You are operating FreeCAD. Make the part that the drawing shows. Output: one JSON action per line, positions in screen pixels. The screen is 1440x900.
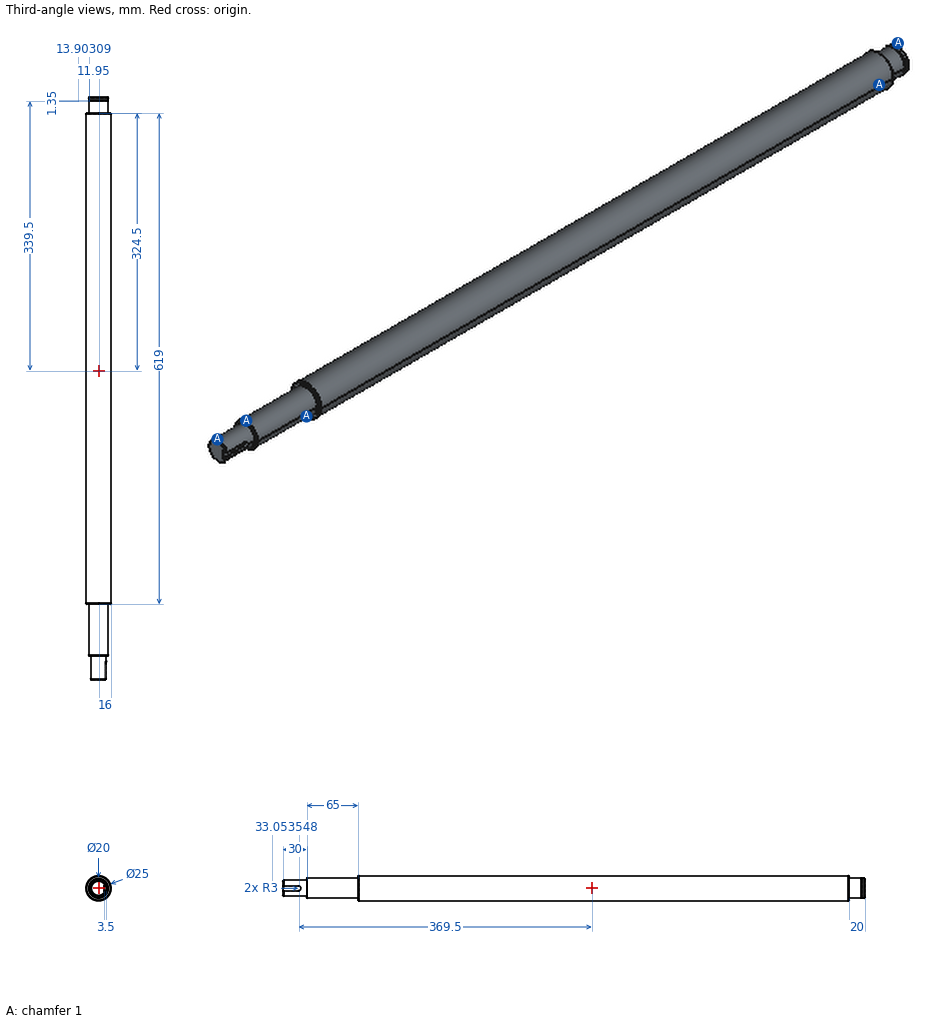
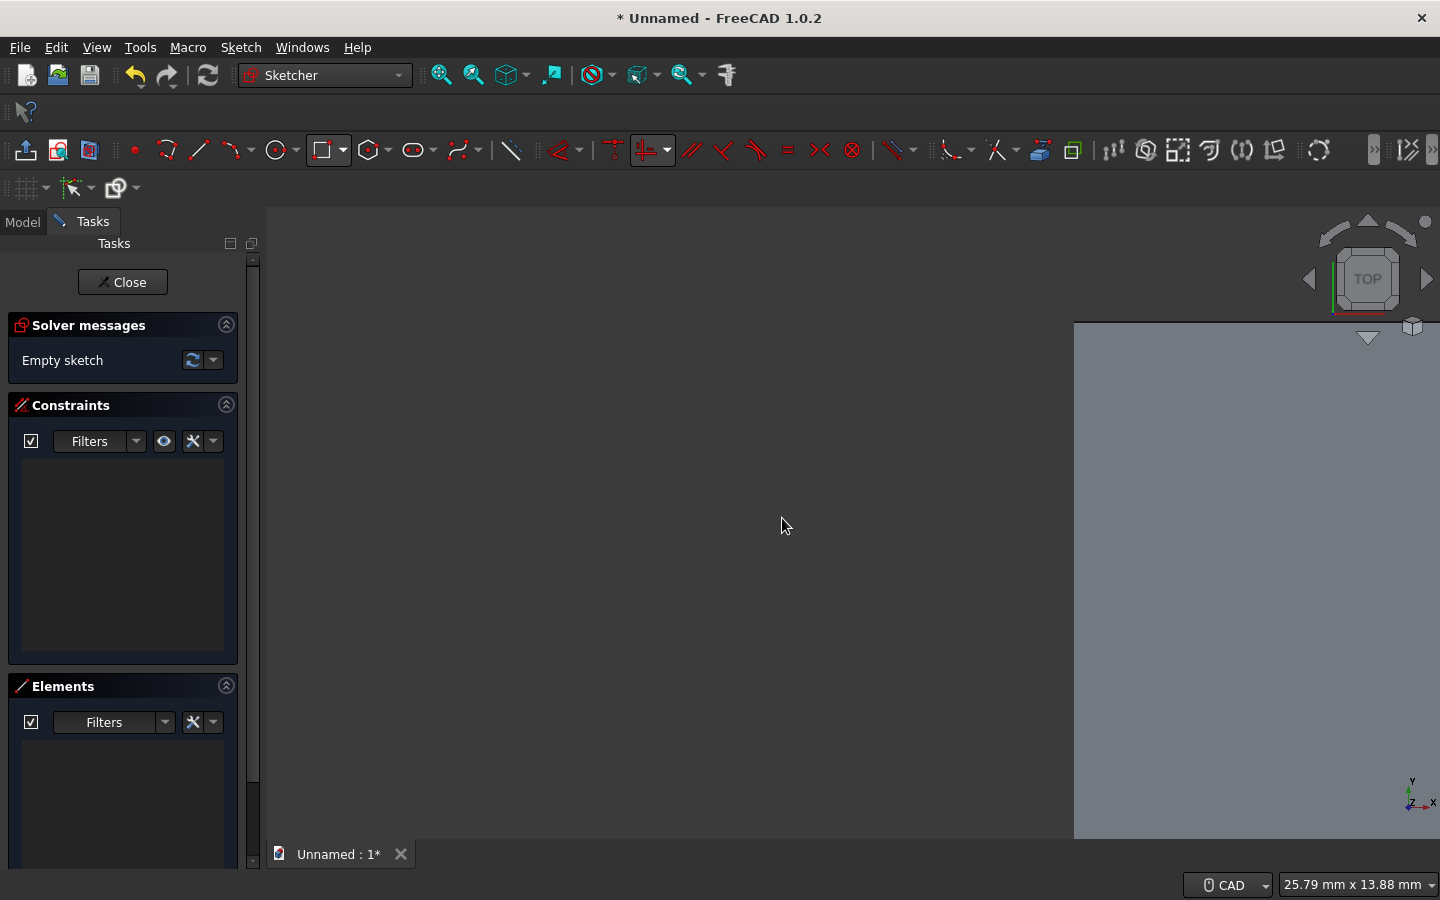
{"action": "left_click", "coordinate": [322, 150]}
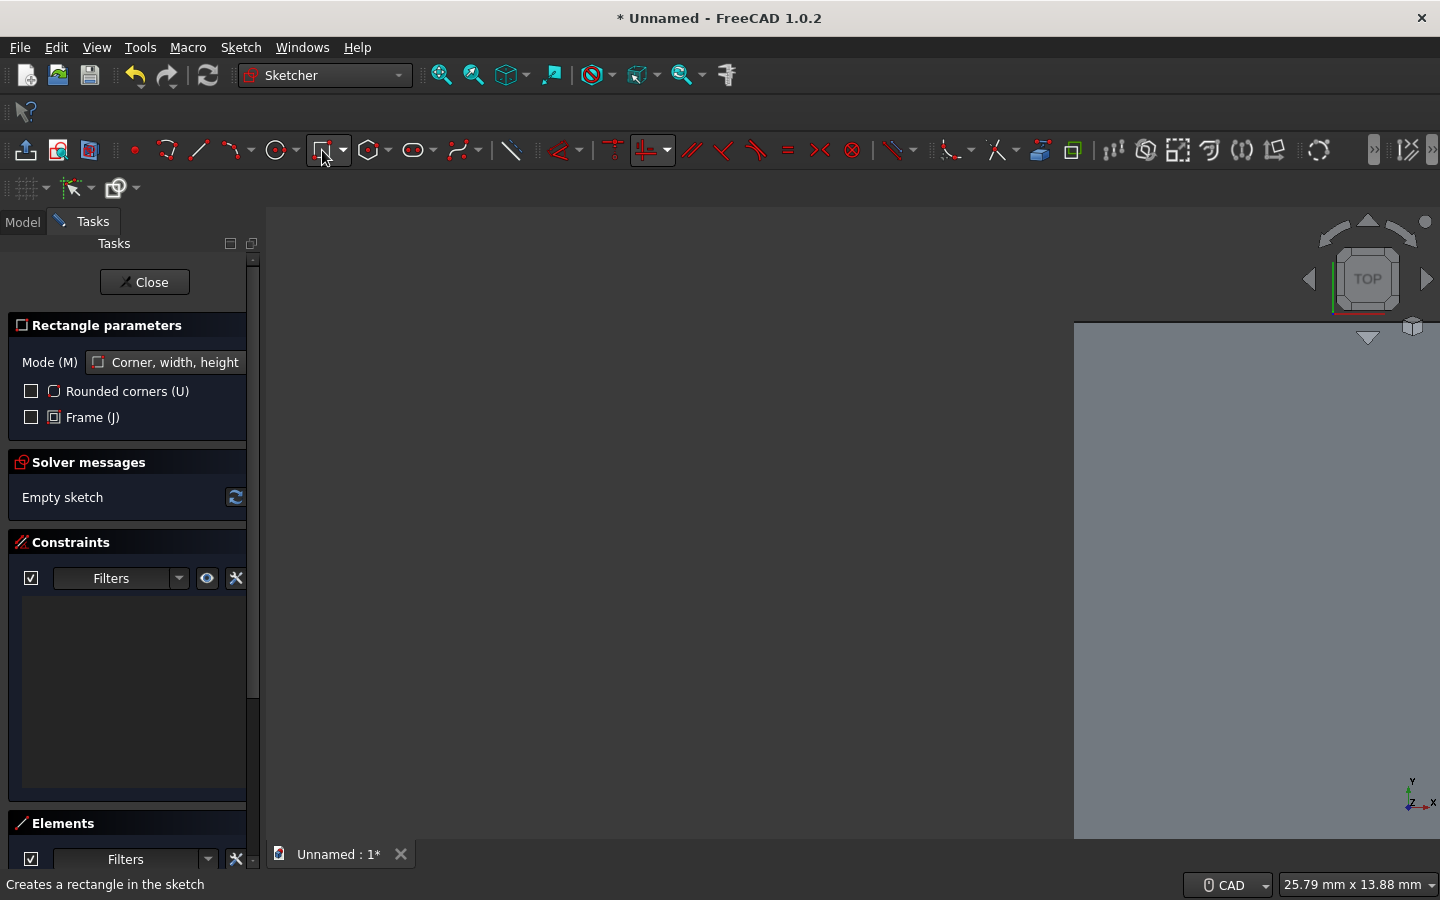
{"action": "left_click", "coordinate": [466, 488]}
{"action": "mouse_move", "coordinate": [1099, 549]}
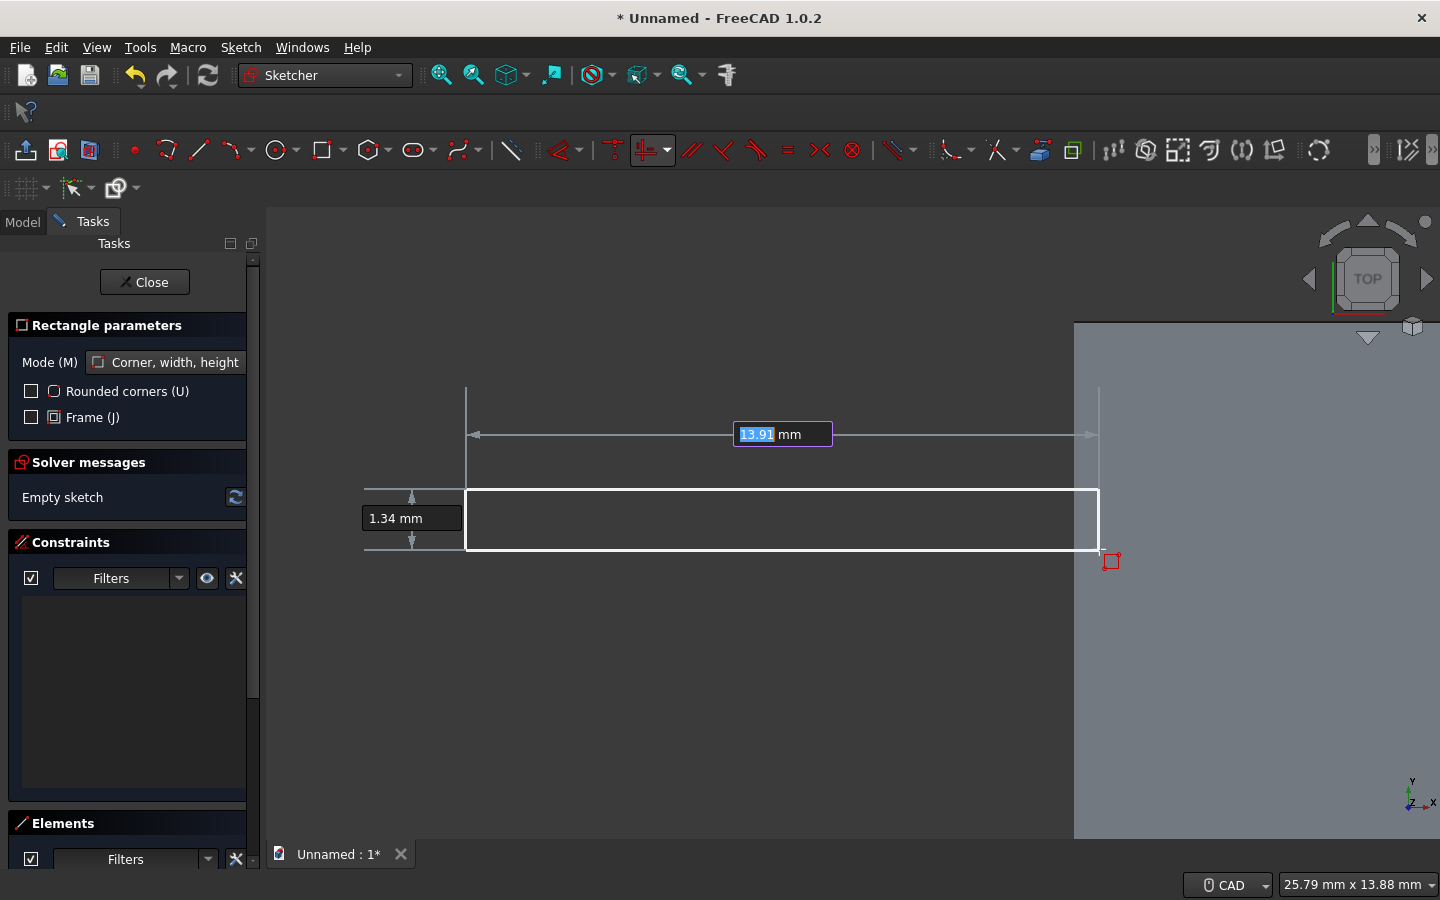
{"action": "type", "text": "13.90309"}
{"action": "key", "text": "Tab"}
{"action": "type", "text": "1.35"}
{"action": "key", "text": "Return"}
{"action": "key", "text": "Escape"}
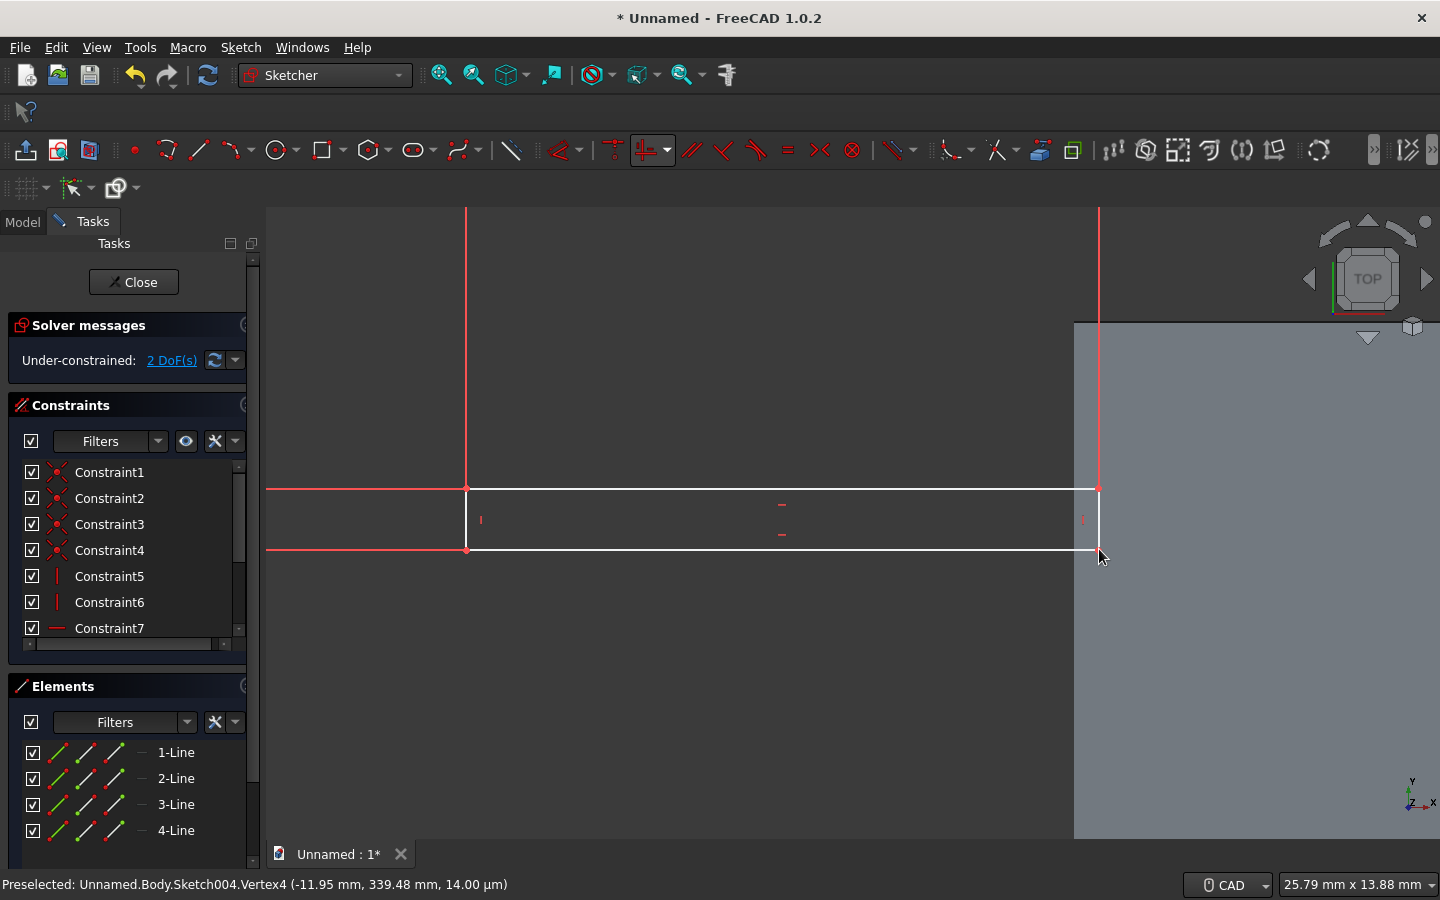
{"action": "left_click", "coordinate": [558, 150]}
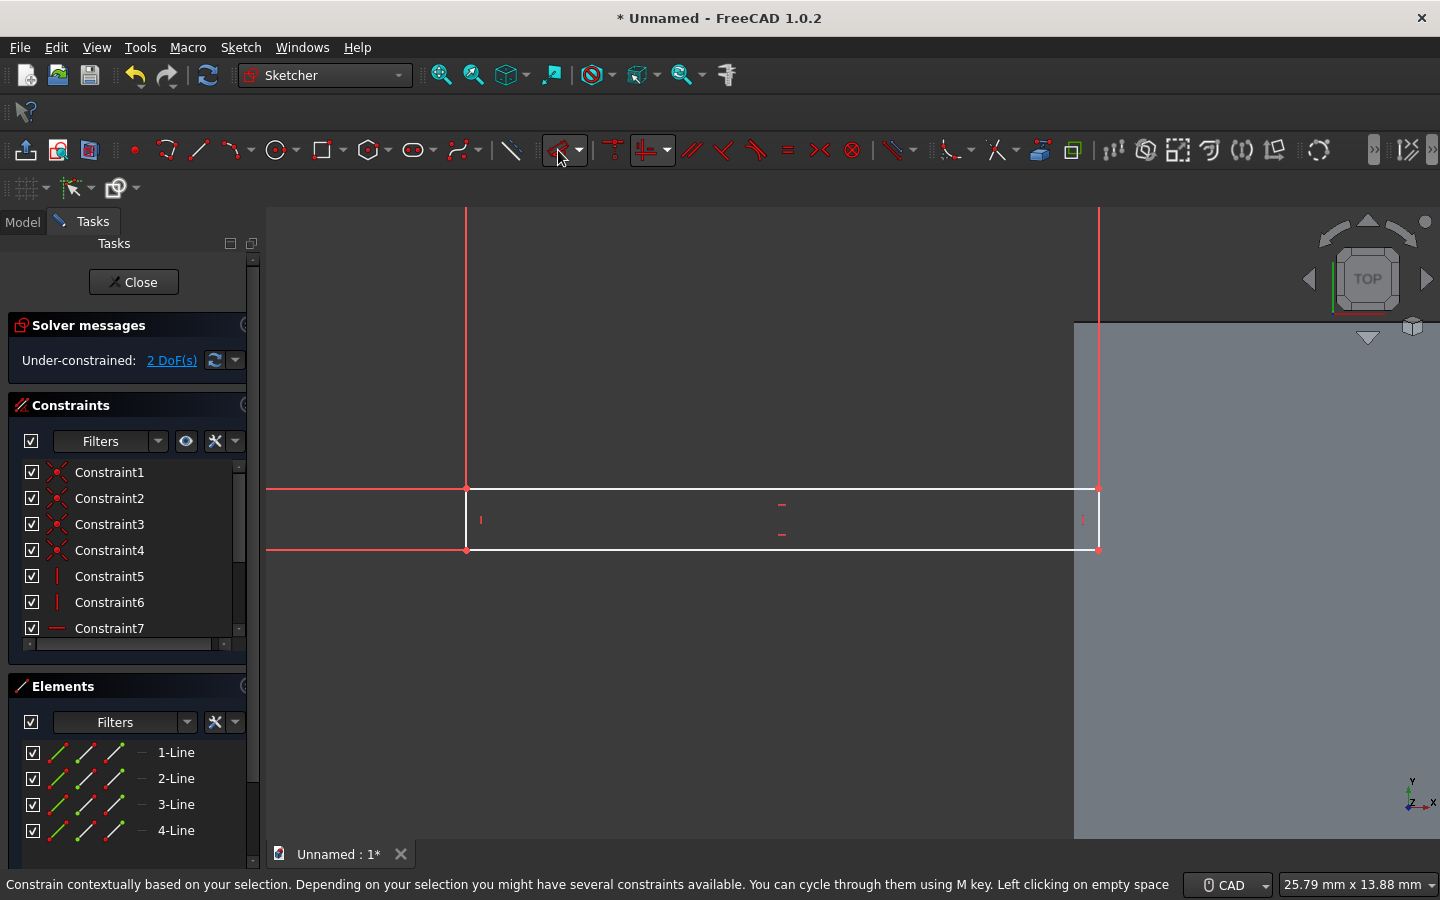
{"action": "left_click", "coordinate": [466, 550]}
{"action": "left_click", "coordinate": [432, 681]}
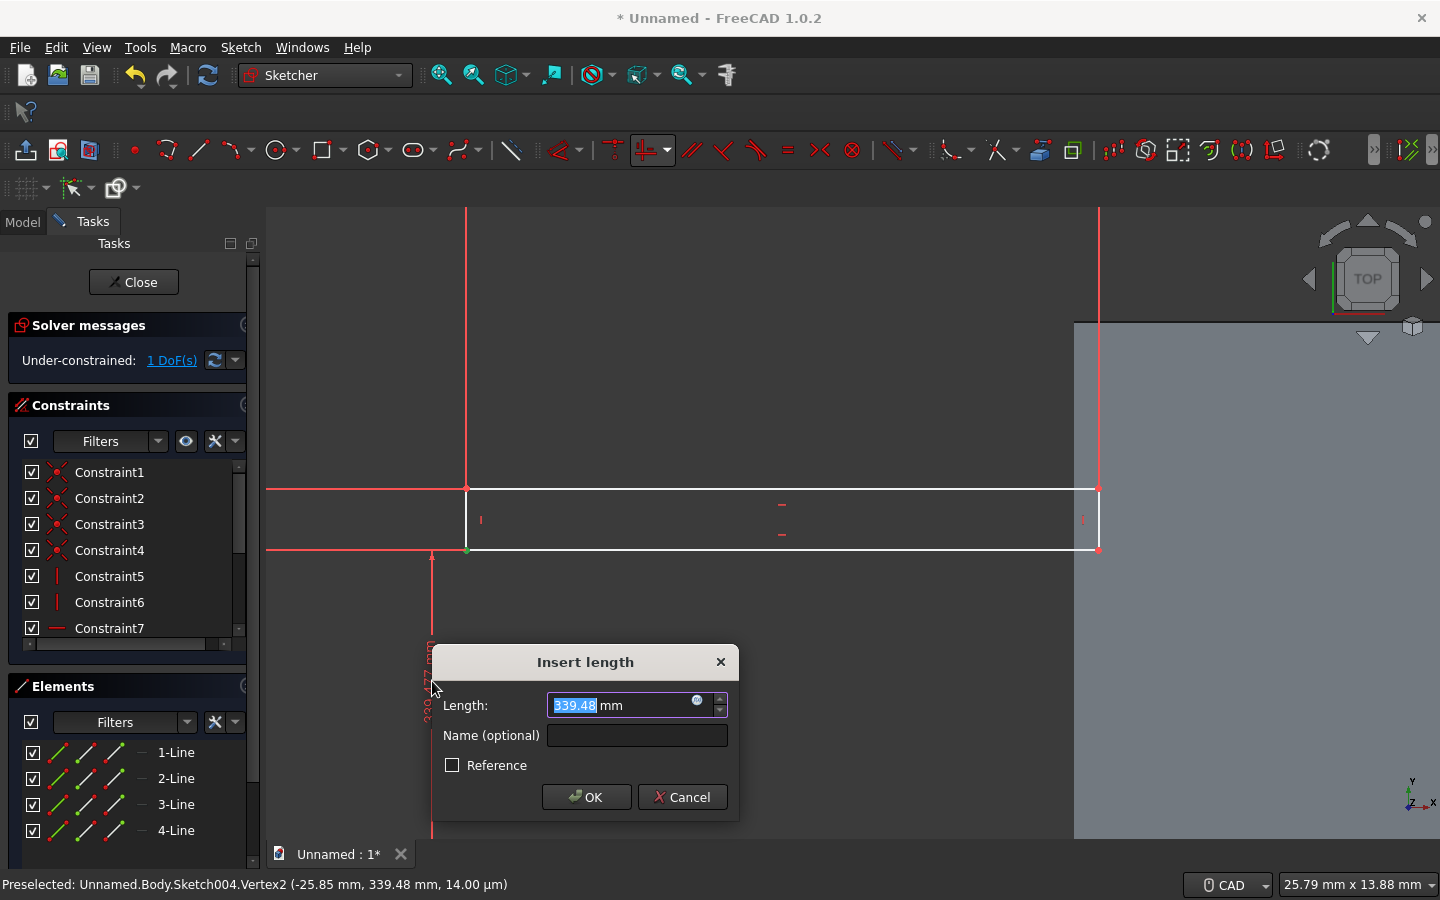
{"action": "type", "text": "339.5"}
{"action": "key", "text": "Return"}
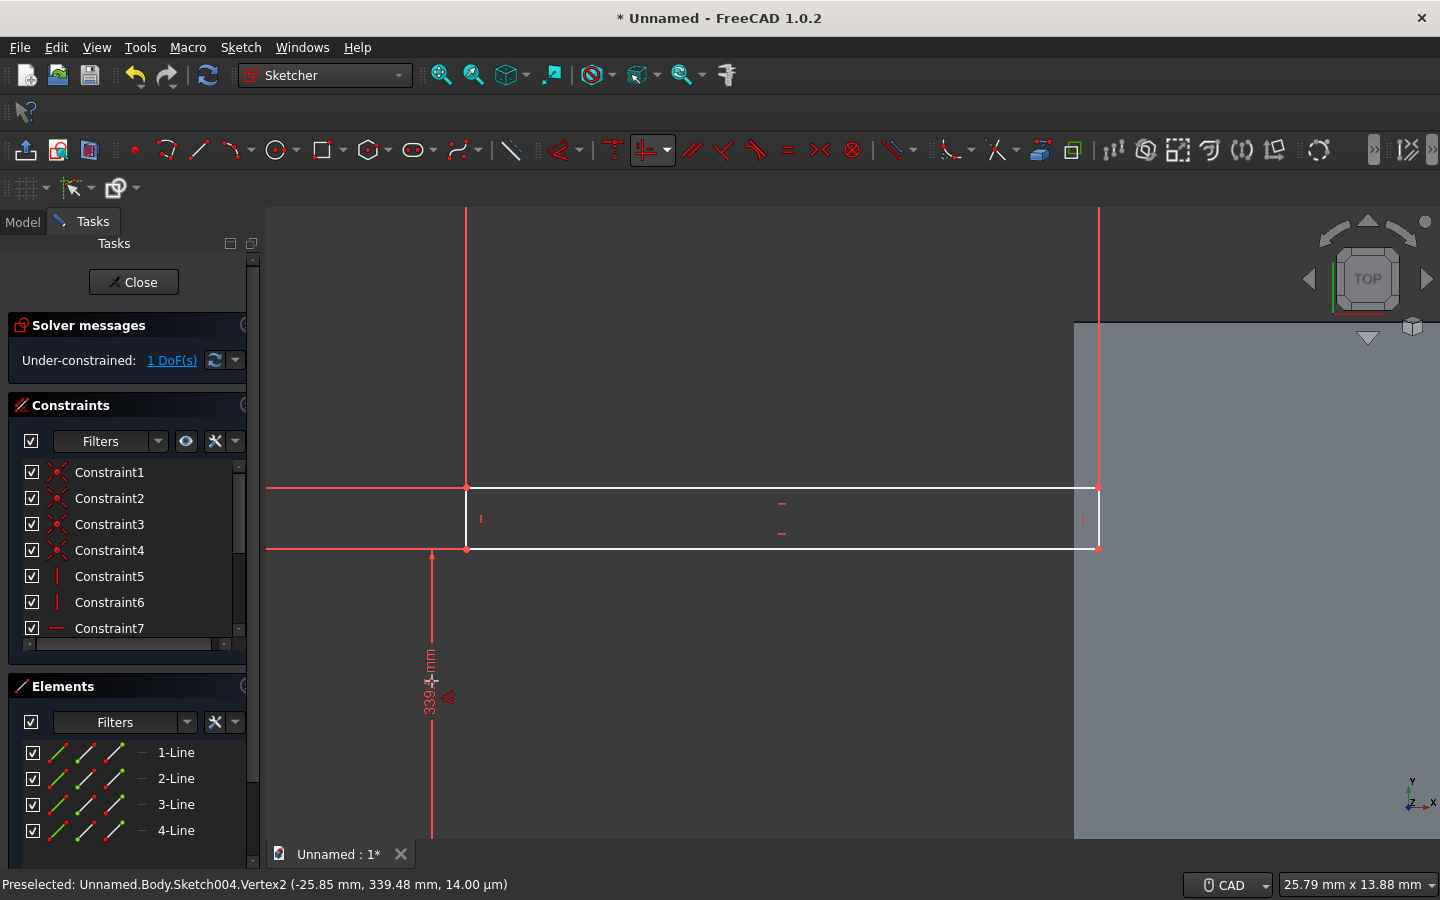
{"action": "left_click", "coordinate": [1099, 549]}
{"action": "left_click", "coordinate": [1187, 515]}